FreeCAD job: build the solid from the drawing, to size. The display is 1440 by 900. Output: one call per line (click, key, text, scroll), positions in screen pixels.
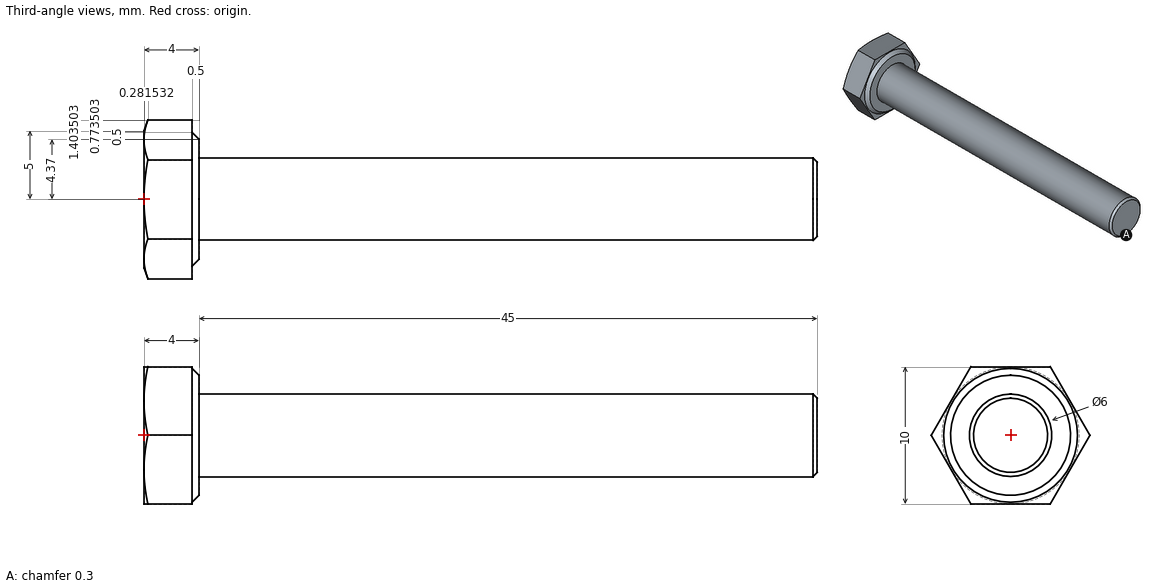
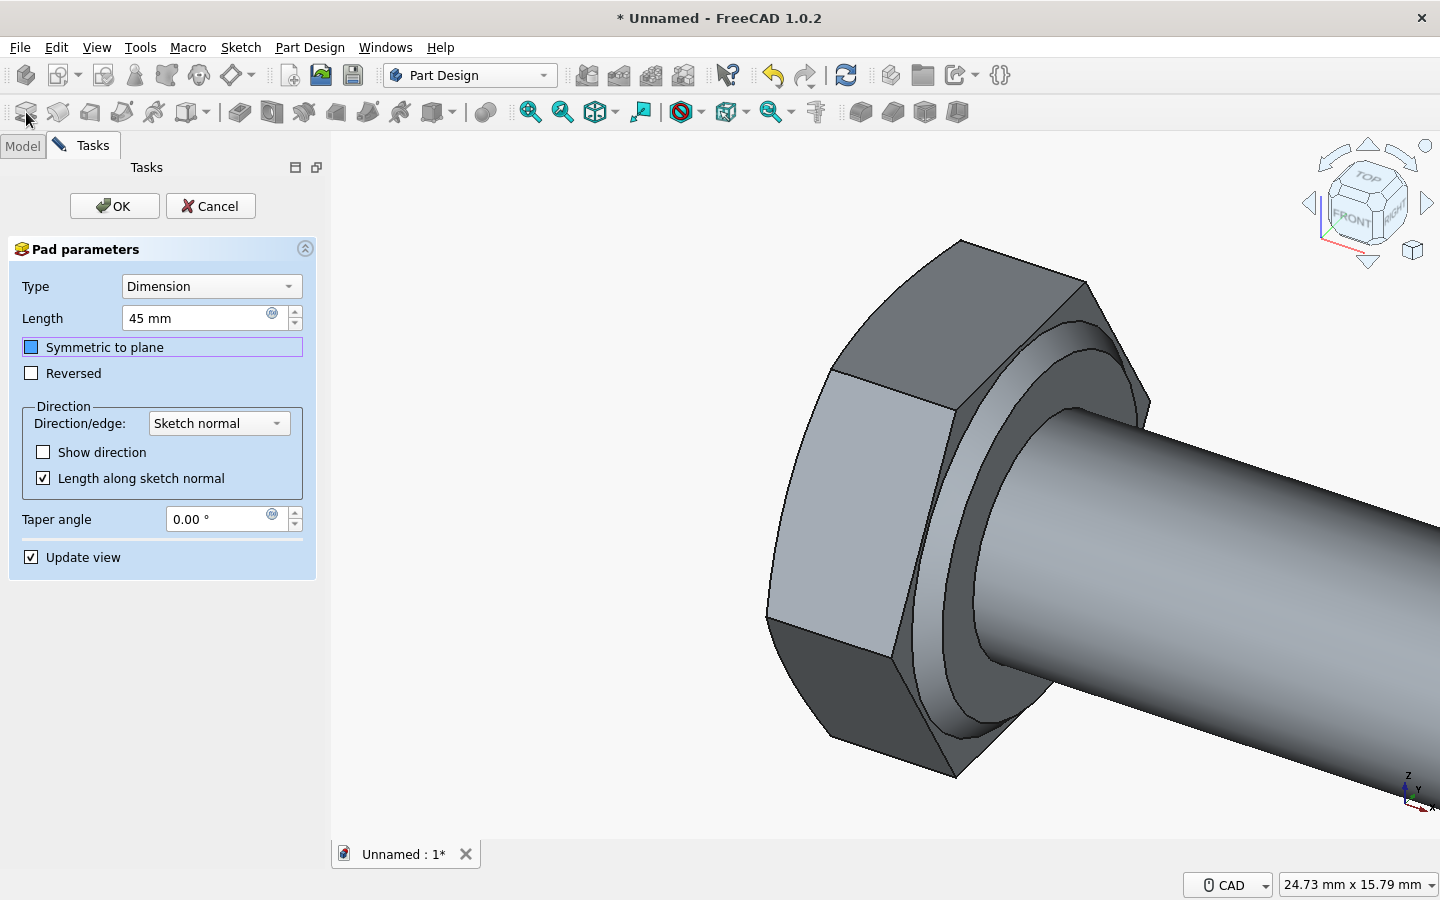
click(115, 206)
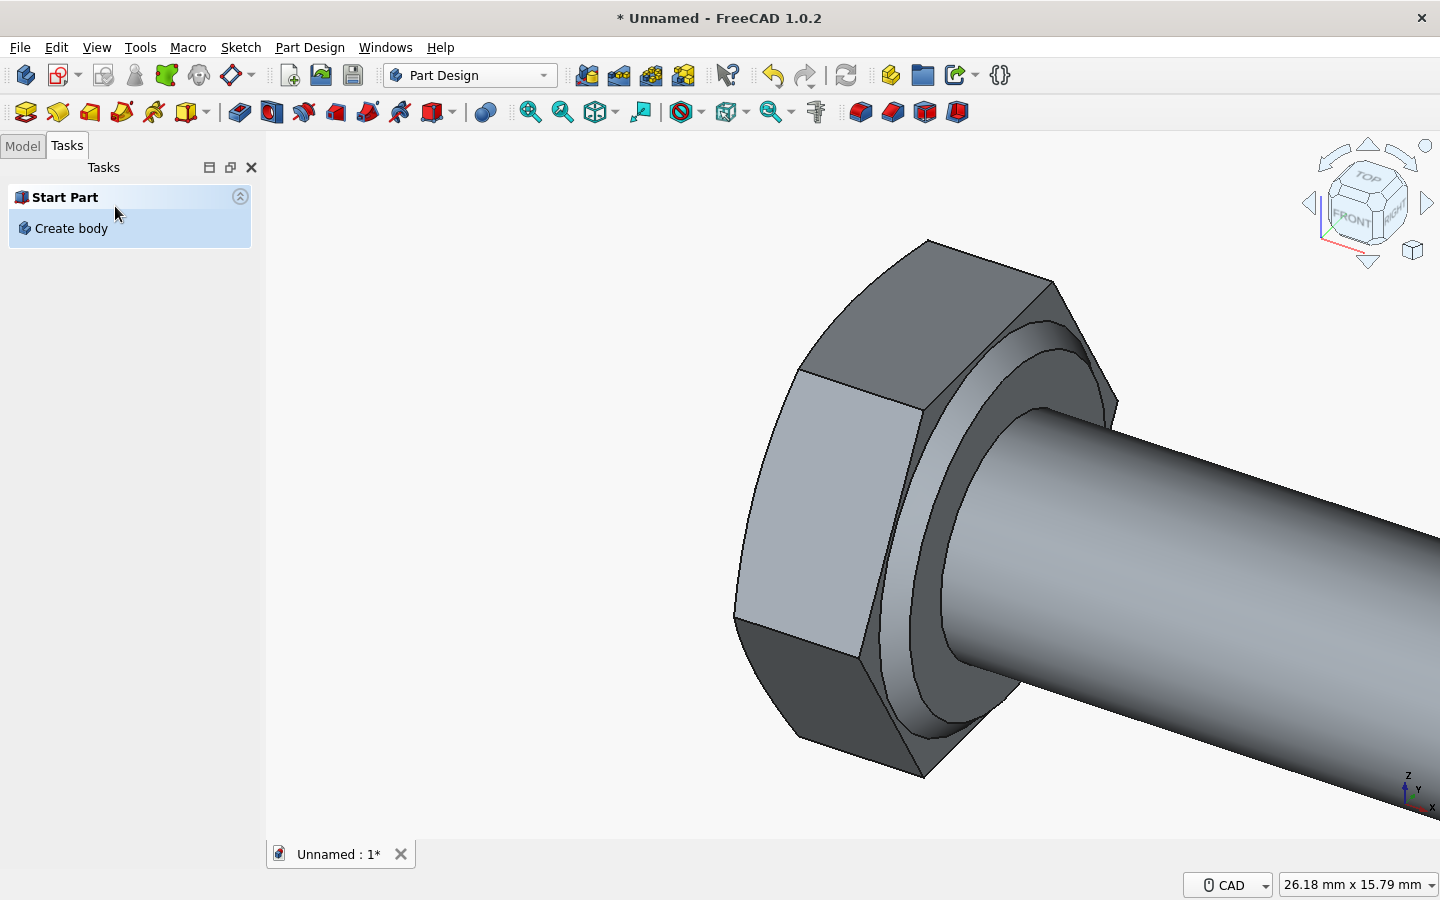
click(532, 112)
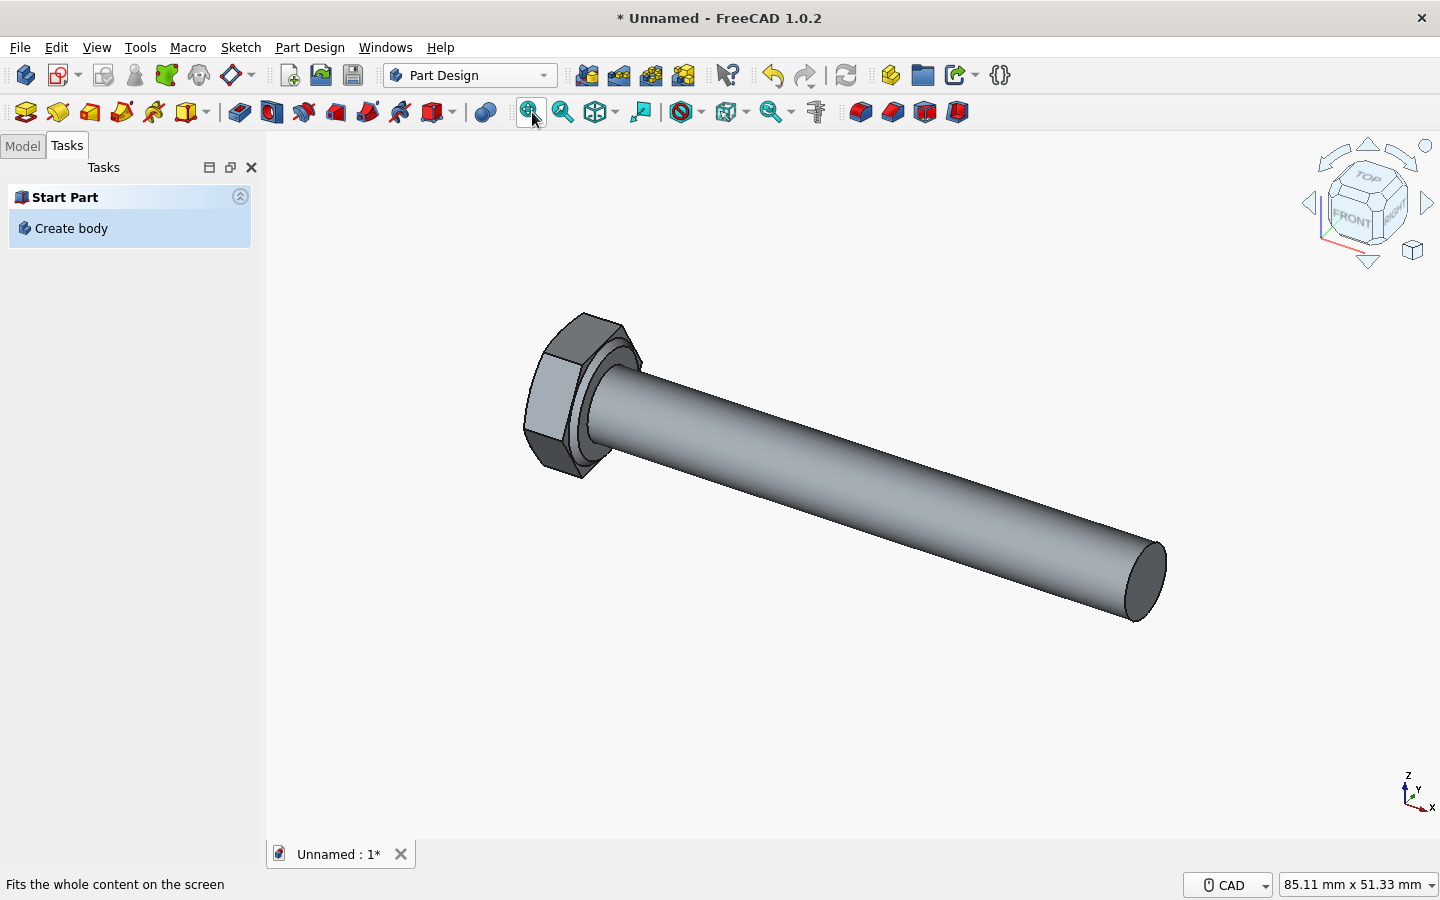
click(1125, 601)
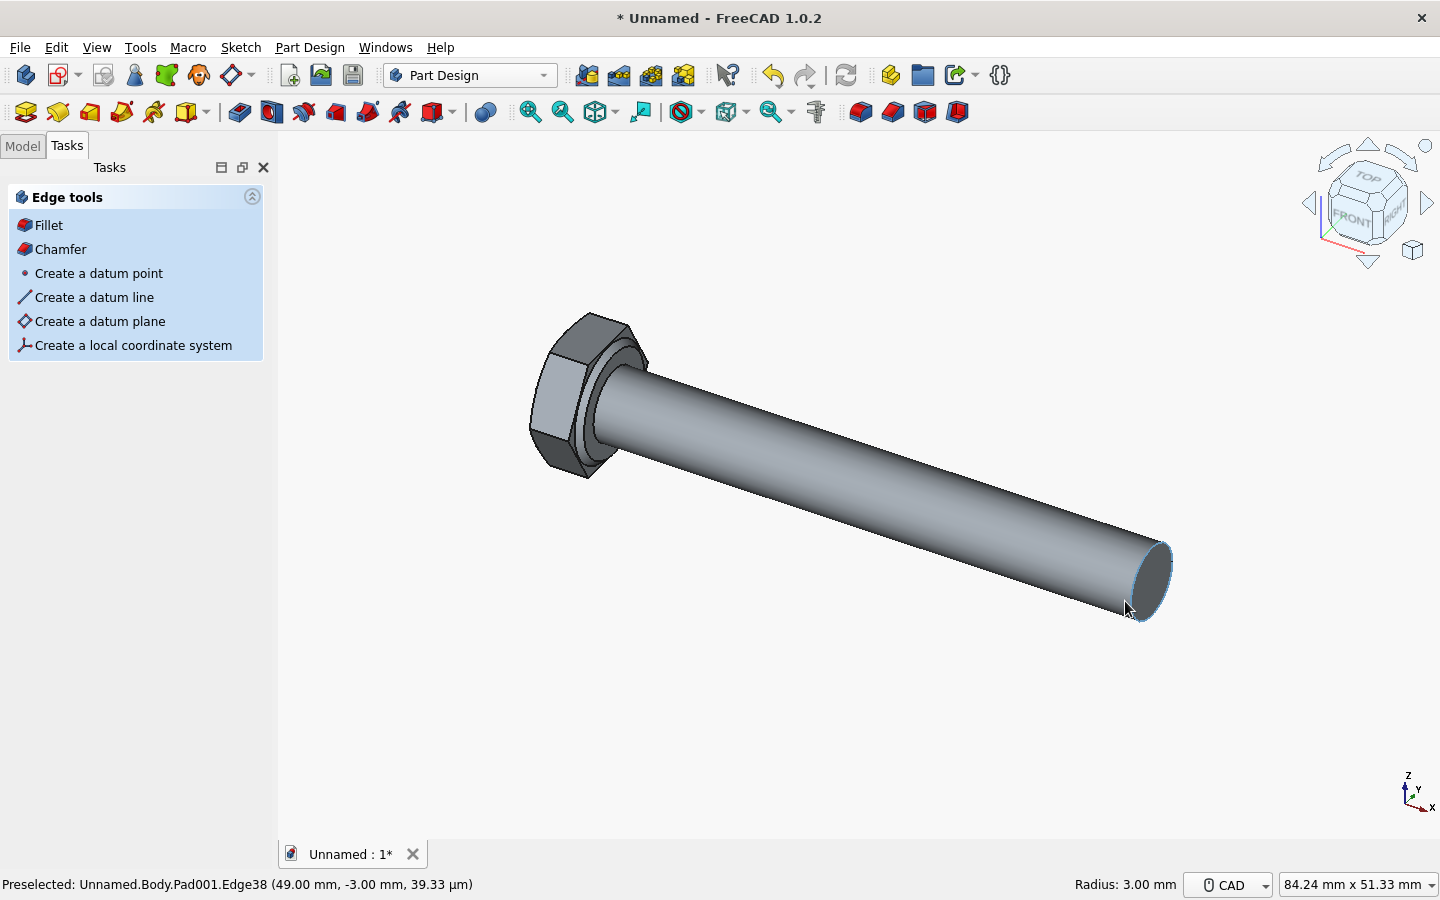
click(894, 112)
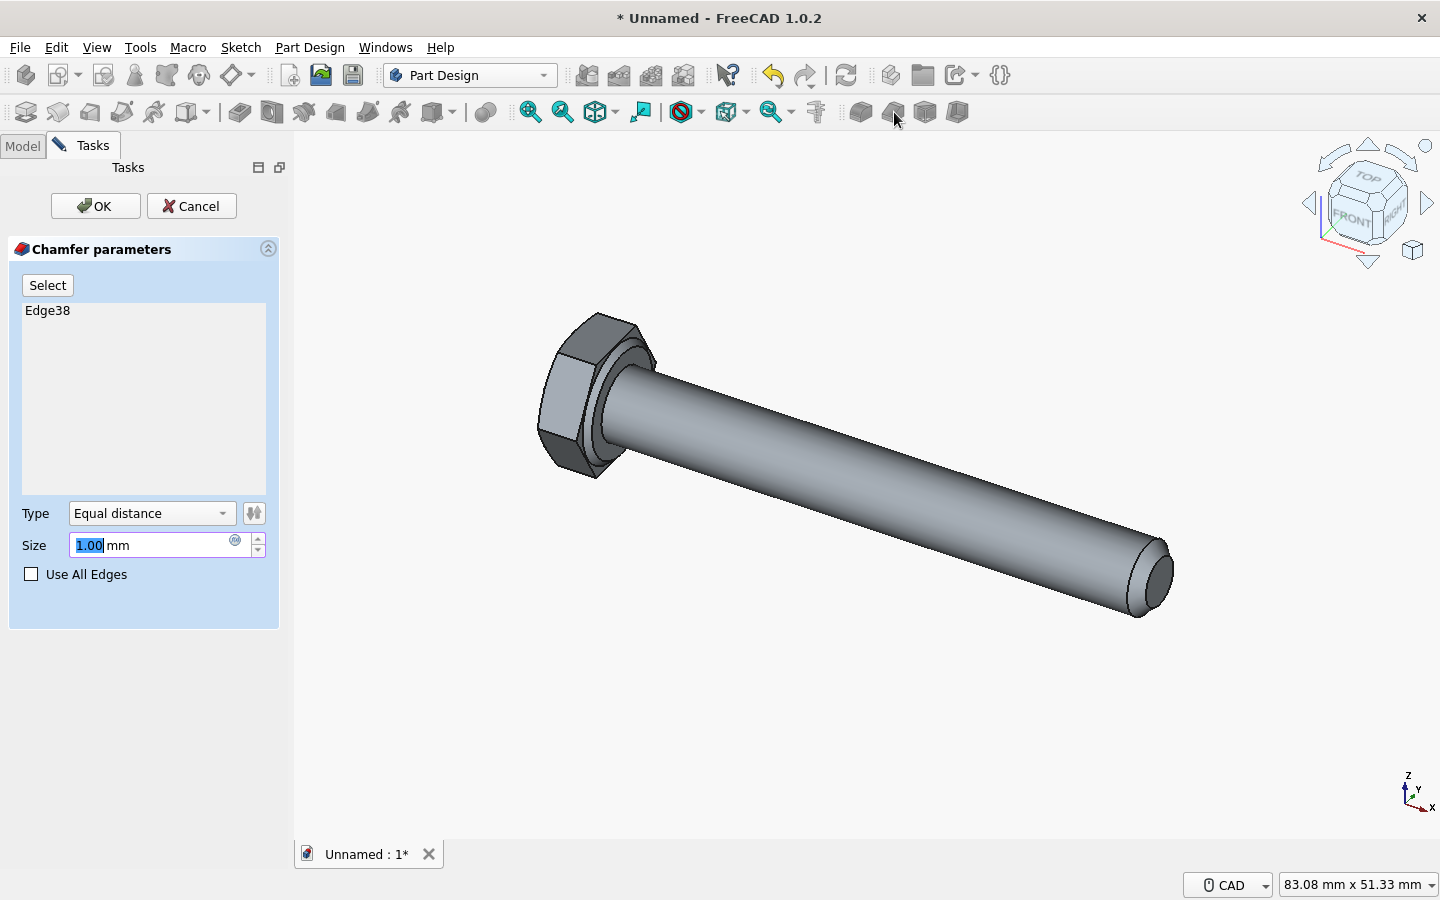
text(0.3)
key(Tab)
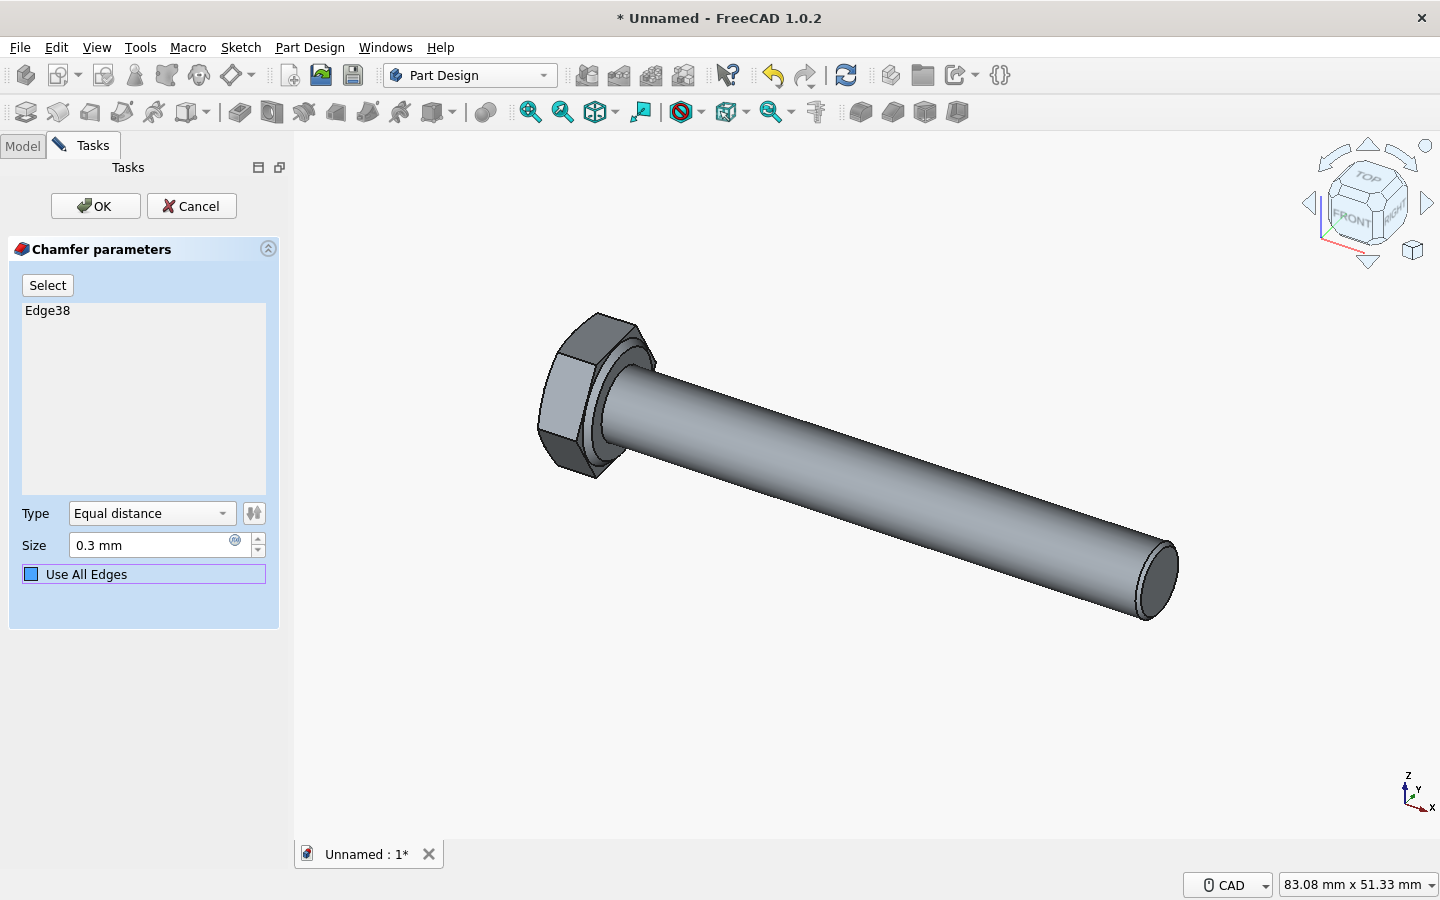
click(96, 206)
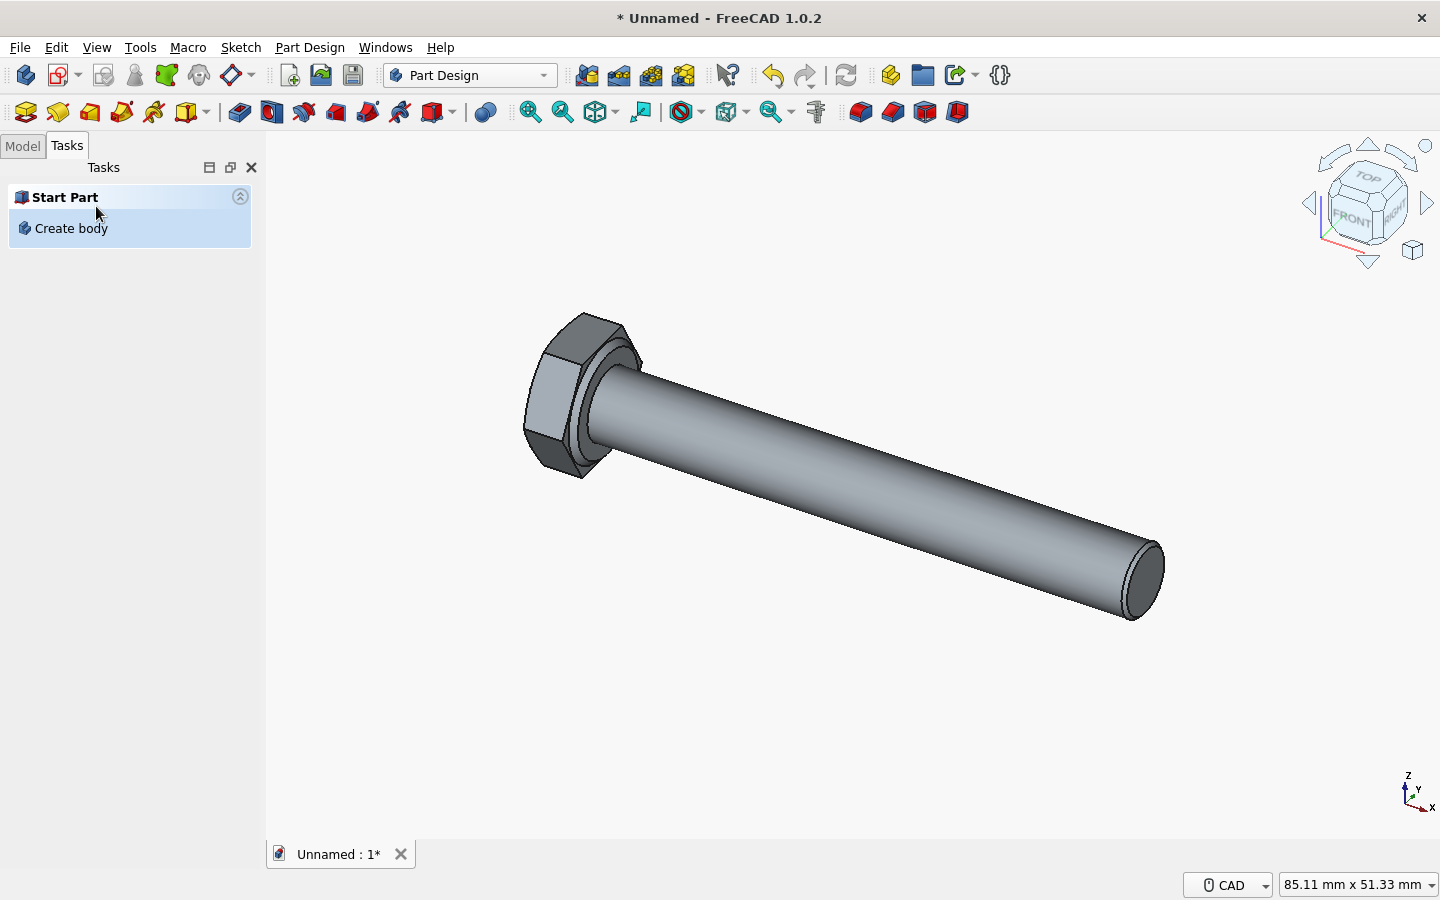
key(0)